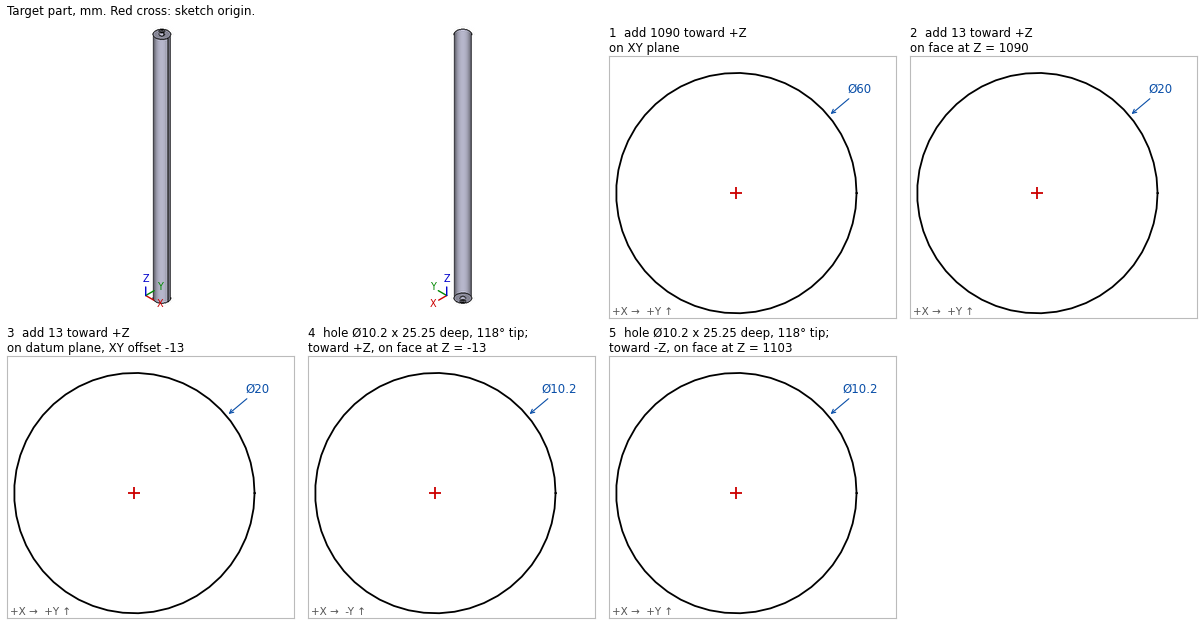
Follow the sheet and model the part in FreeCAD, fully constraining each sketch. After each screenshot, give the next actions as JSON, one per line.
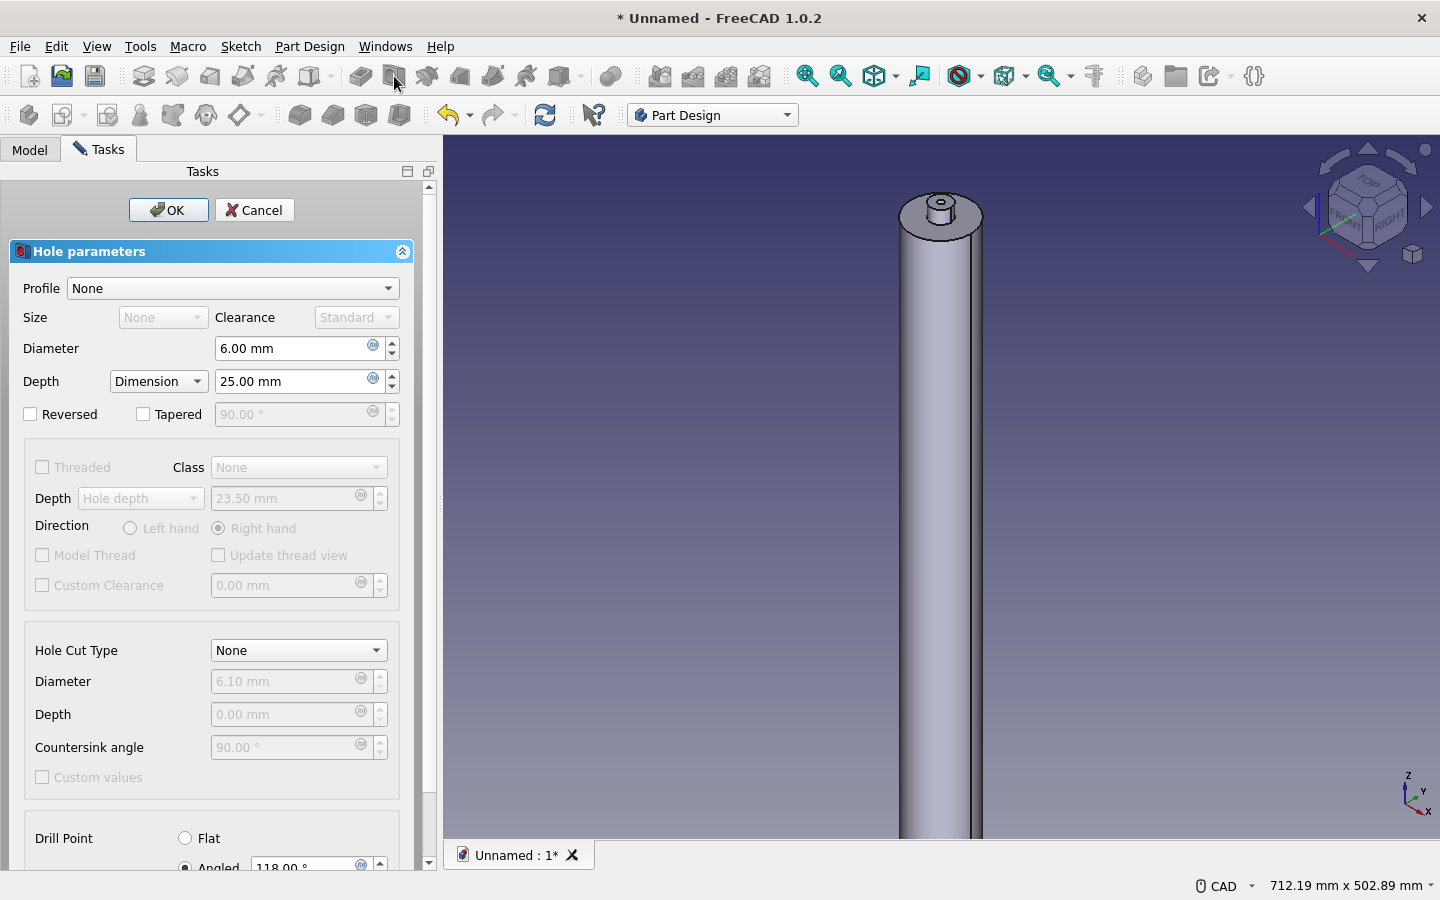
{"action": "triple_click", "coordinate": [300, 348]}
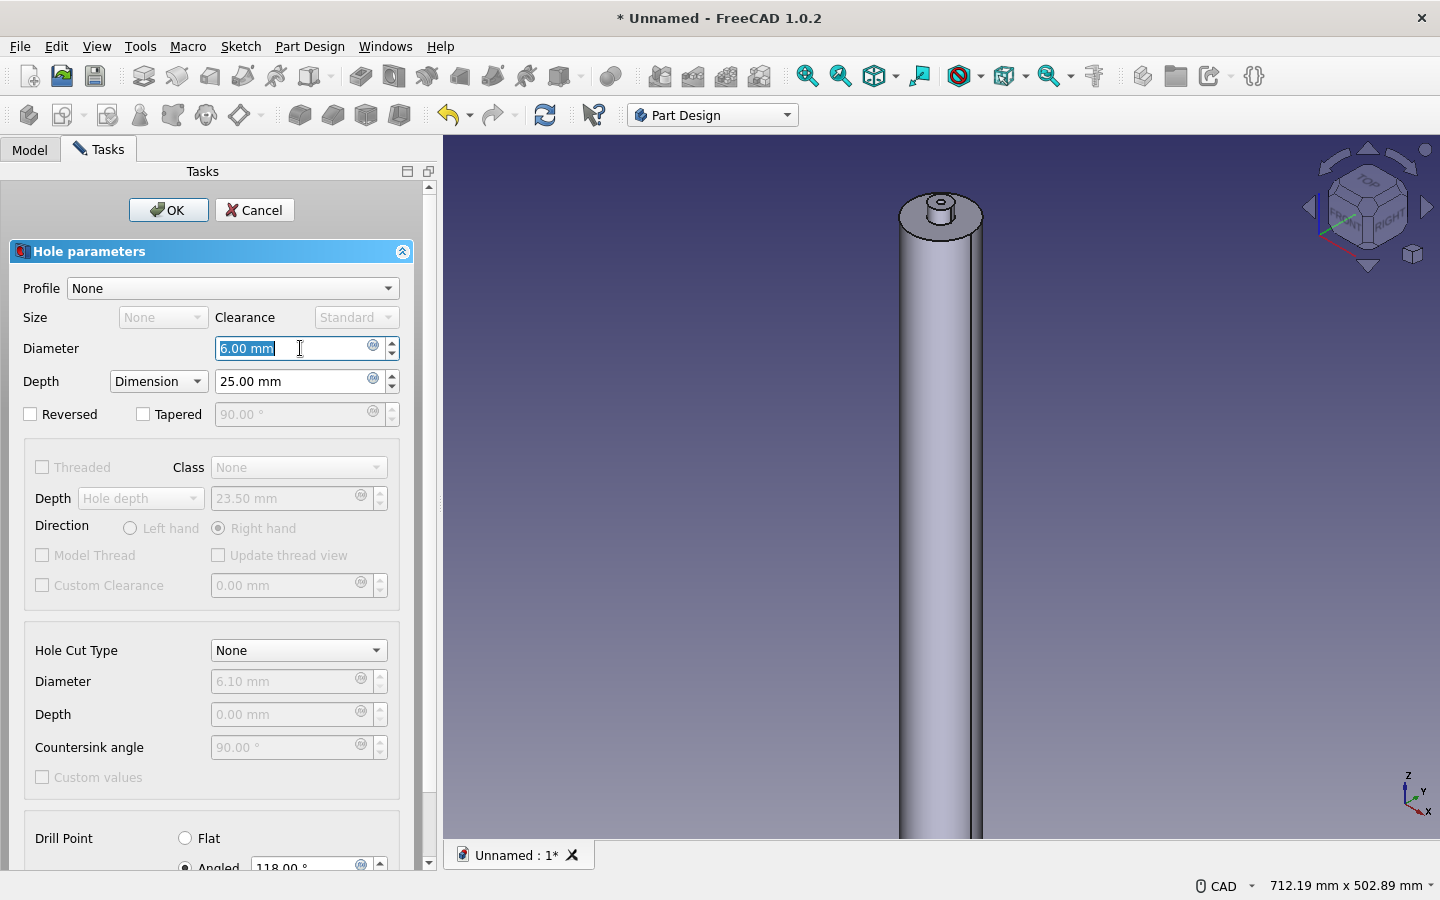
{"action": "type", "text": "10.2"}
{"action": "key", "text": "Tab"}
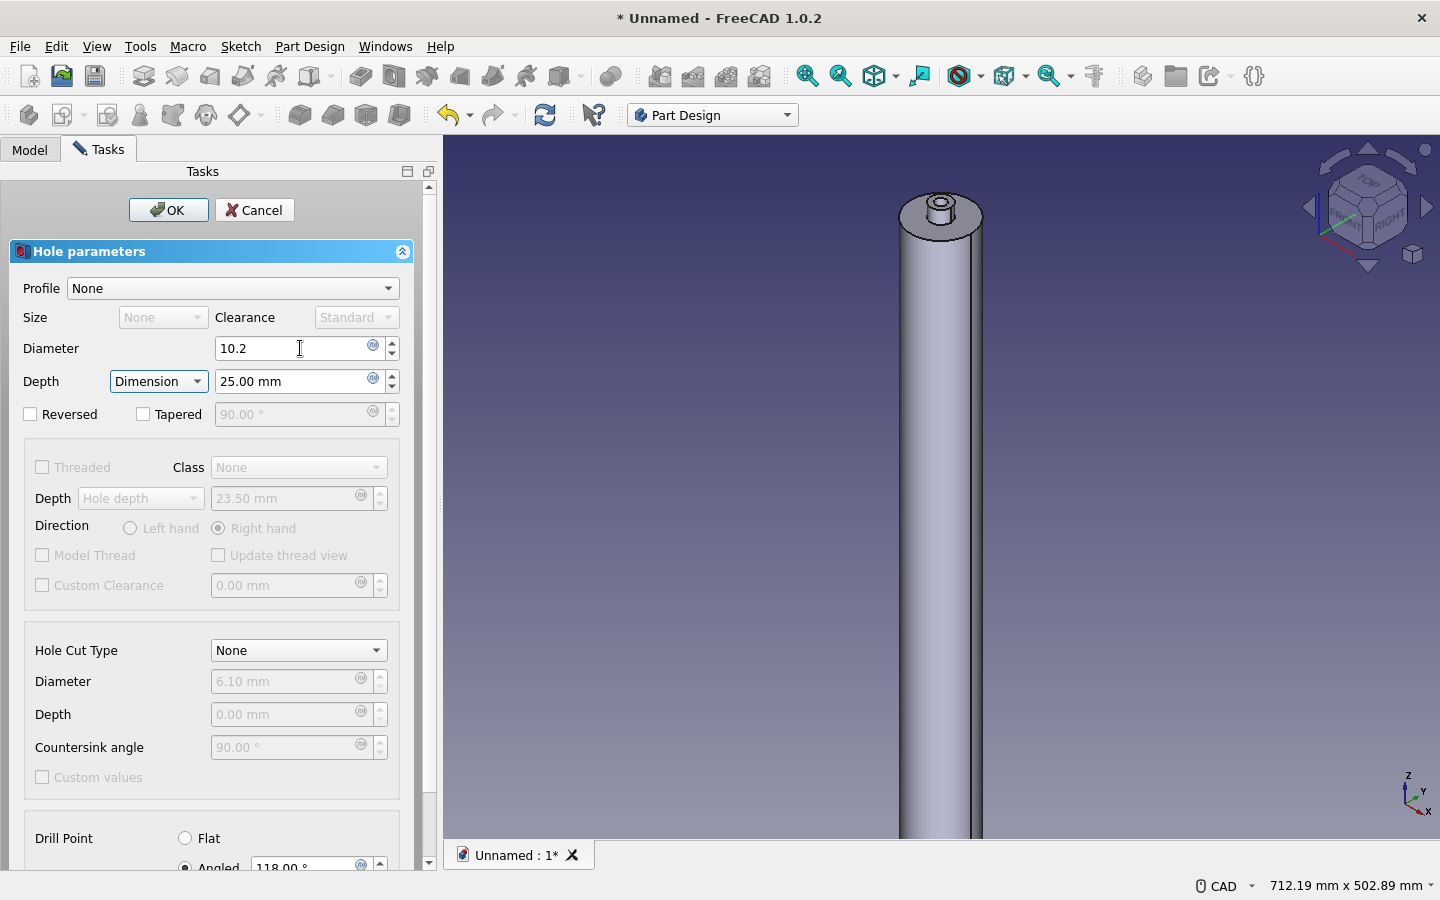
{"action": "triple_click", "coordinate": [300, 382]}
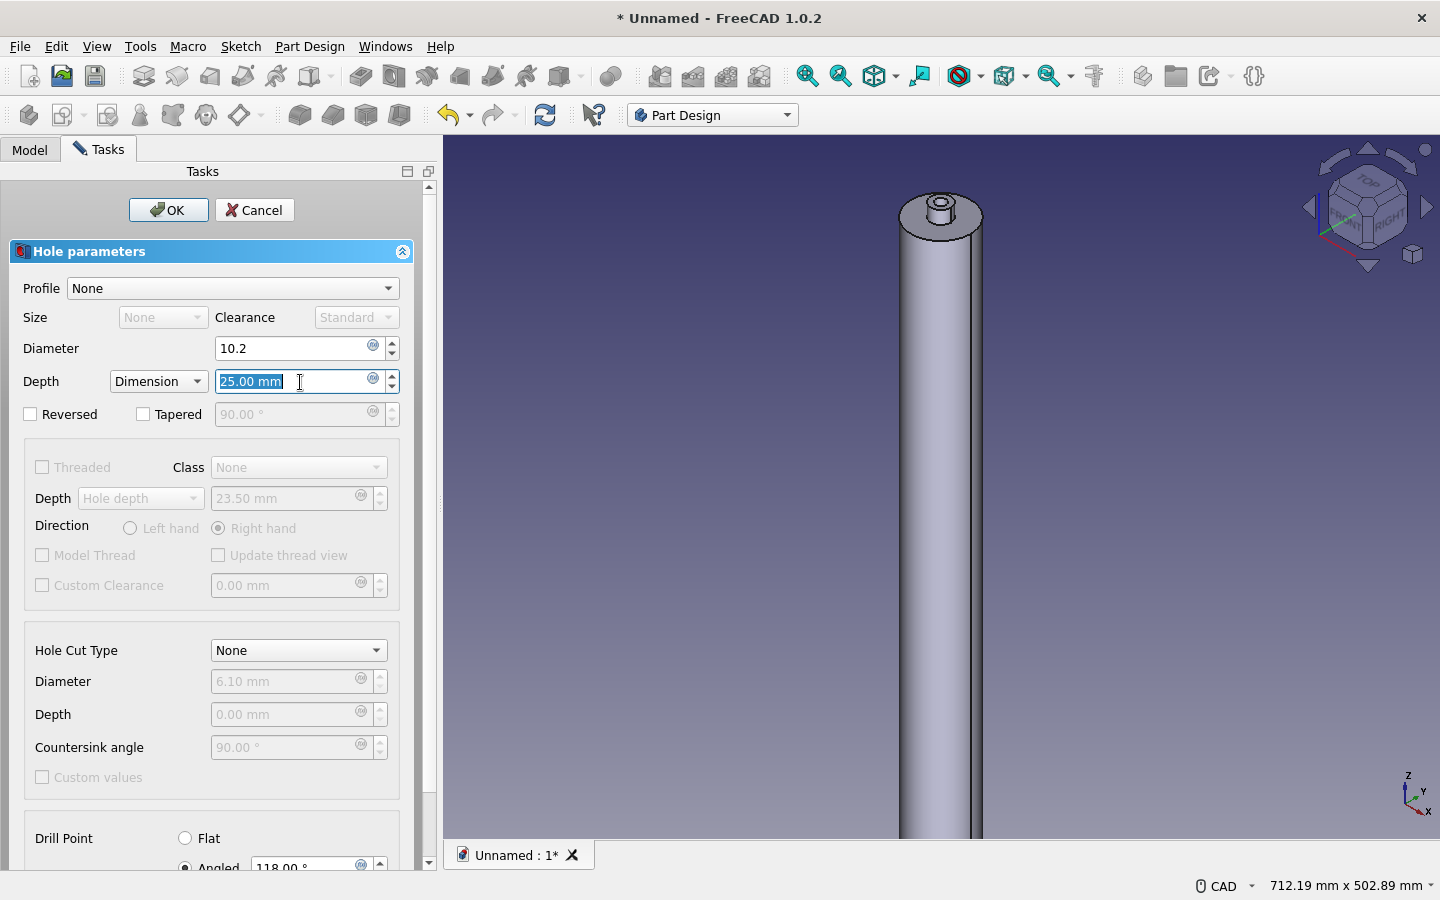
{"action": "type", "text": "25.25"}
{"action": "key", "text": "Tab"}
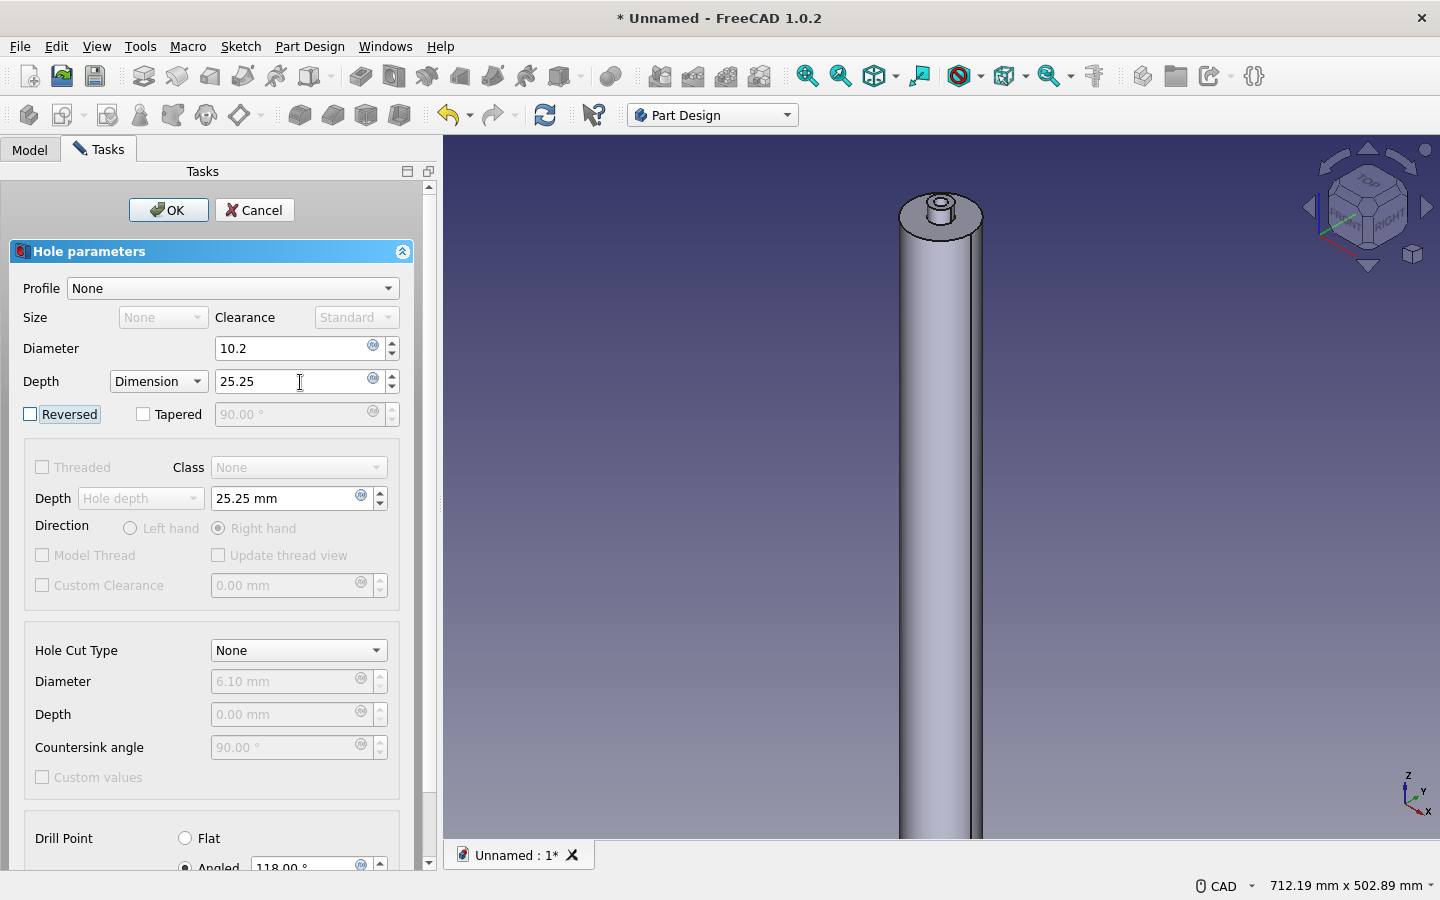
{"action": "left_click", "coordinate": [169, 210]}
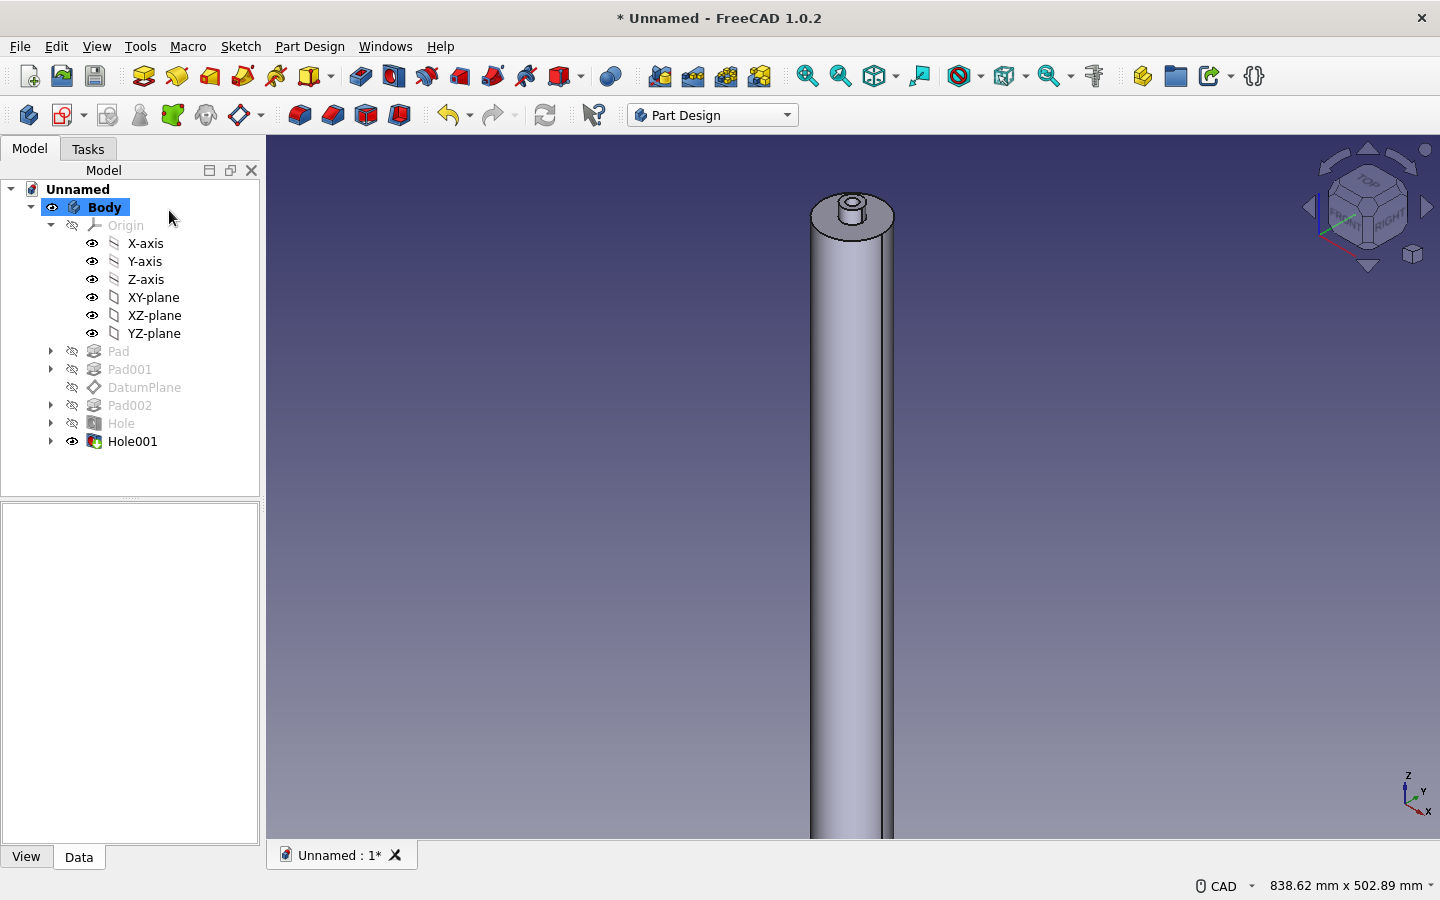
{"action": "key", "text": "v f"}